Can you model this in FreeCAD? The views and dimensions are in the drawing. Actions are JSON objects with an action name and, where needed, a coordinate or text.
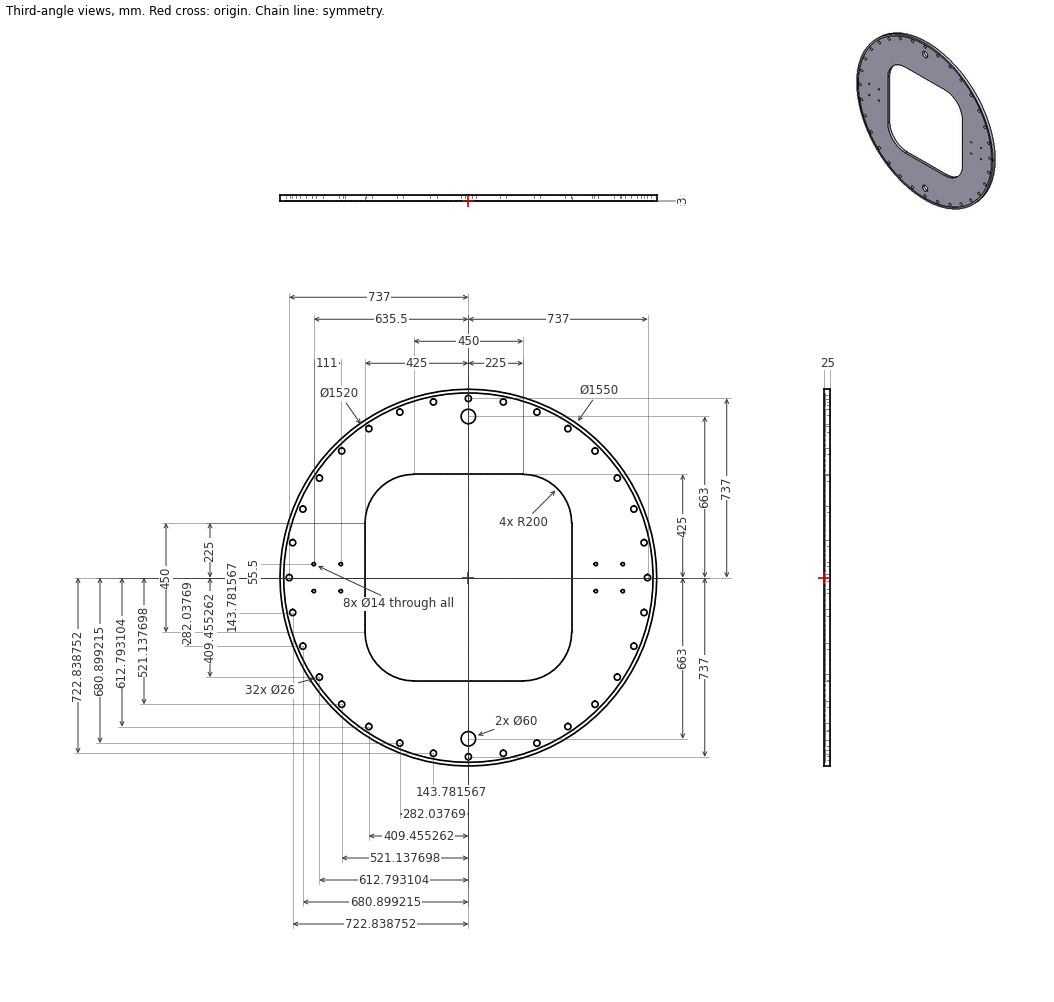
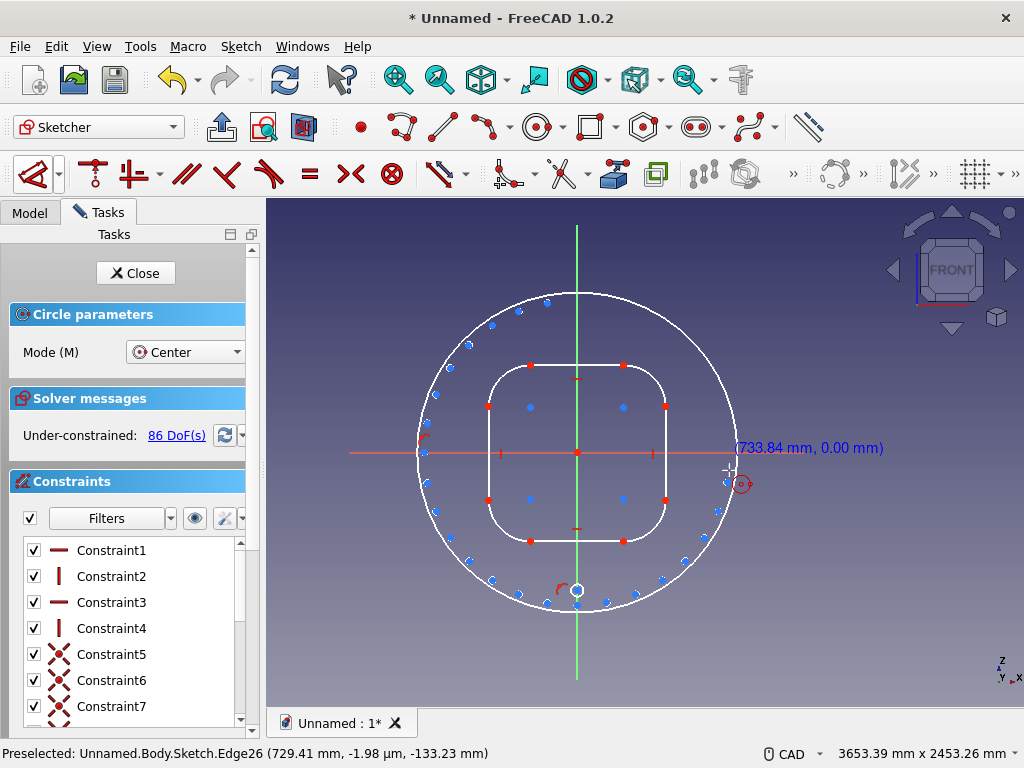
{"action": "scroll", "coordinate": [730, 453], "scroll_direction": "up", "scroll_amount": 4}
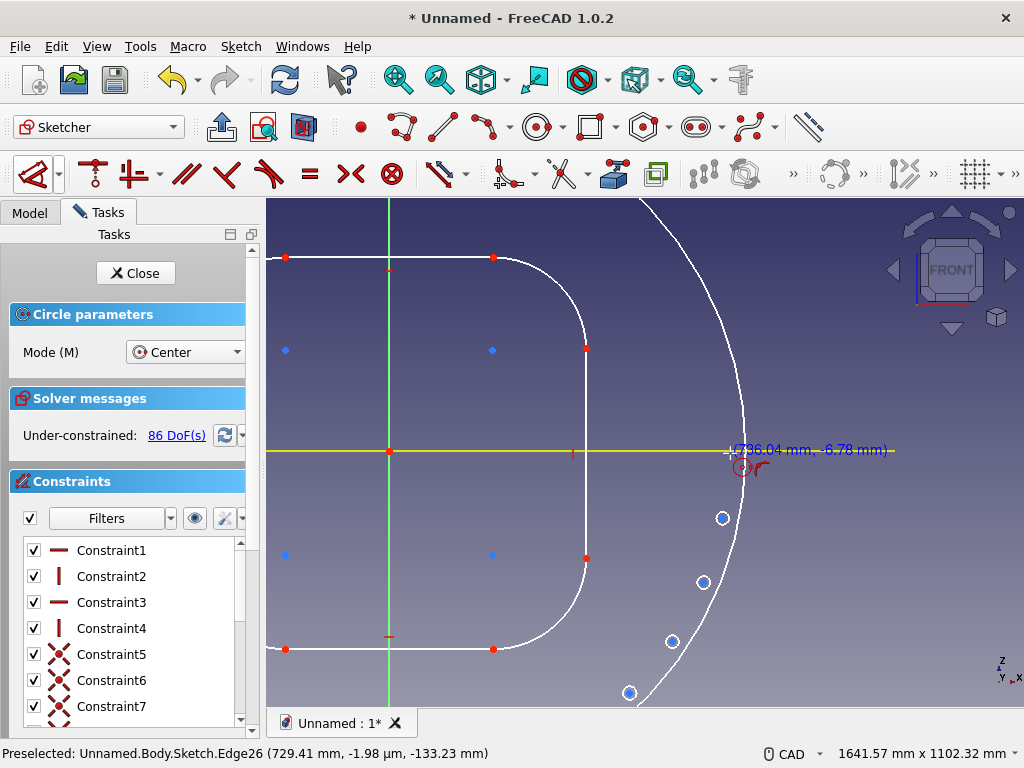
{"action": "left_click", "coordinate": [730, 451]}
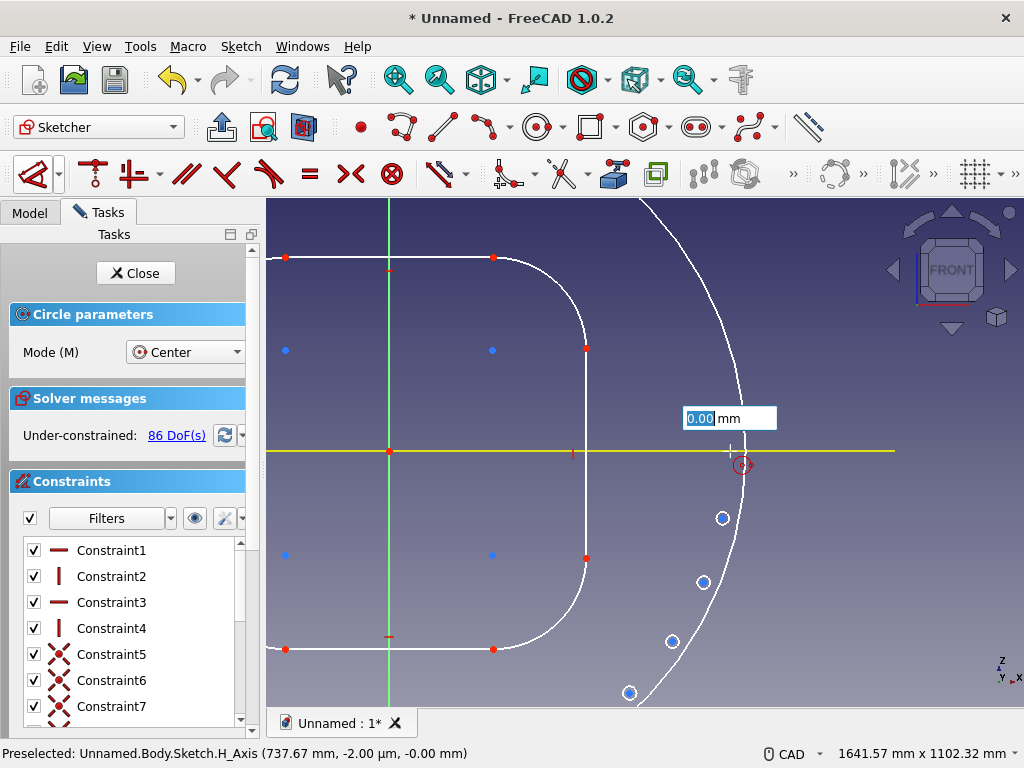
{"action": "scroll", "coordinate": [728, 457], "scroll_direction": "up", "scroll_amount": 6}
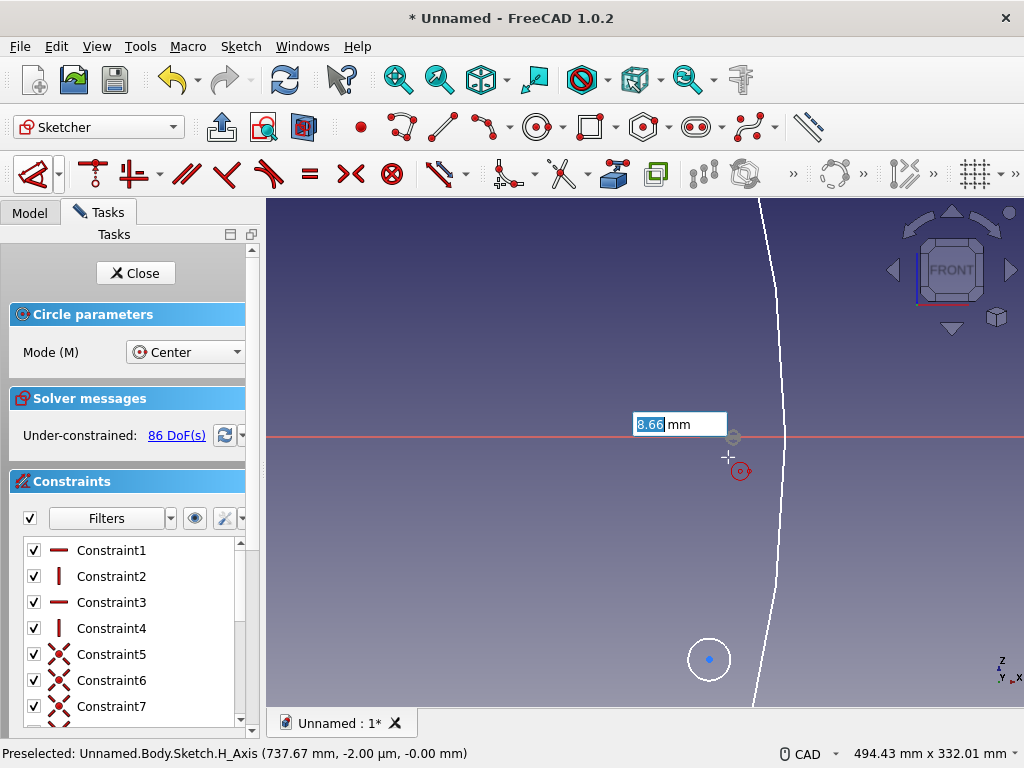
{"action": "left_click", "coordinate": [725, 456]}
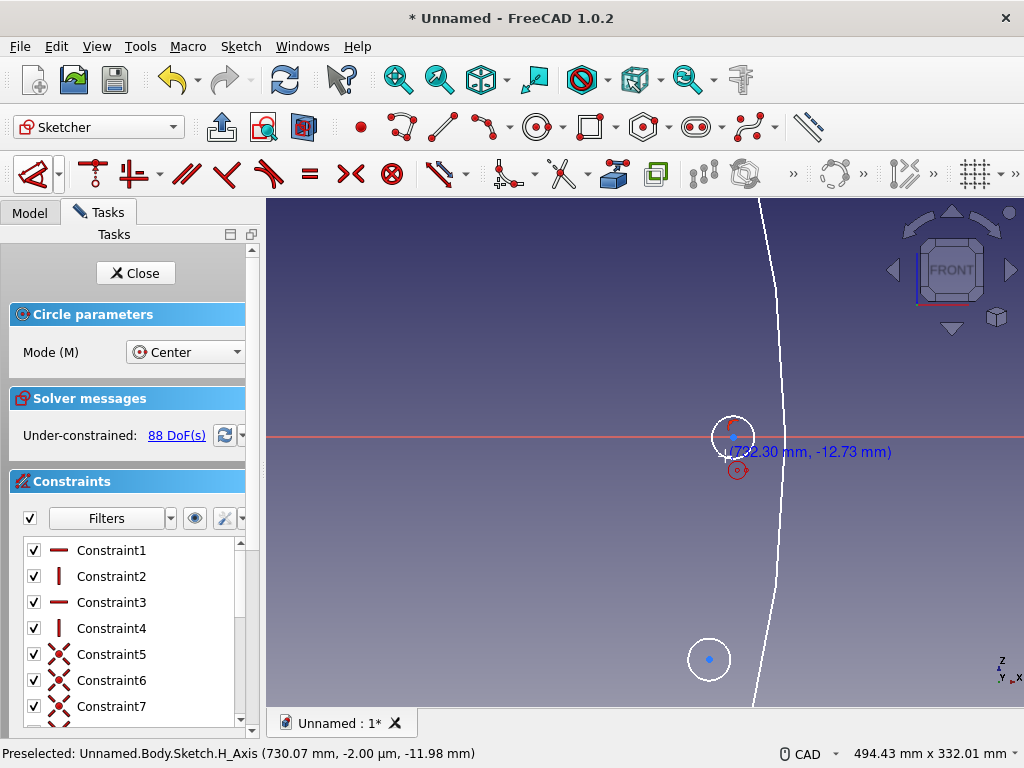
{"action": "scroll", "coordinate": [729, 455], "scroll_direction": "down", "scroll_amount": 10}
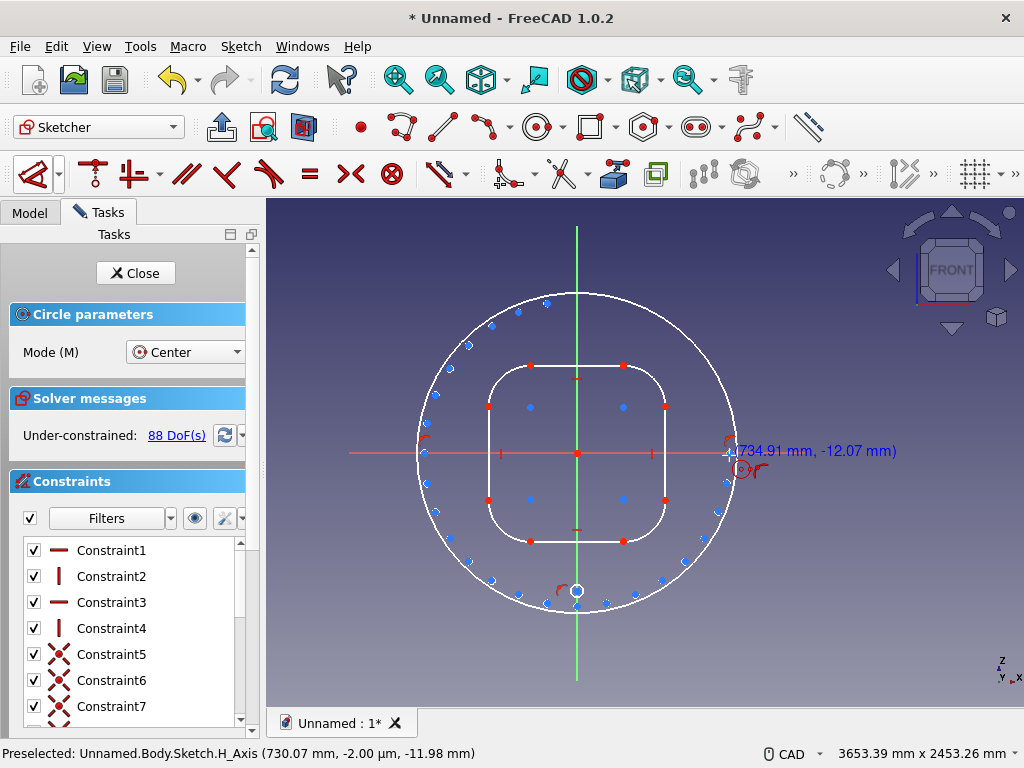
{"action": "scroll", "coordinate": [577, 316], "scroll_direction": "up", "scroll_amount": 7}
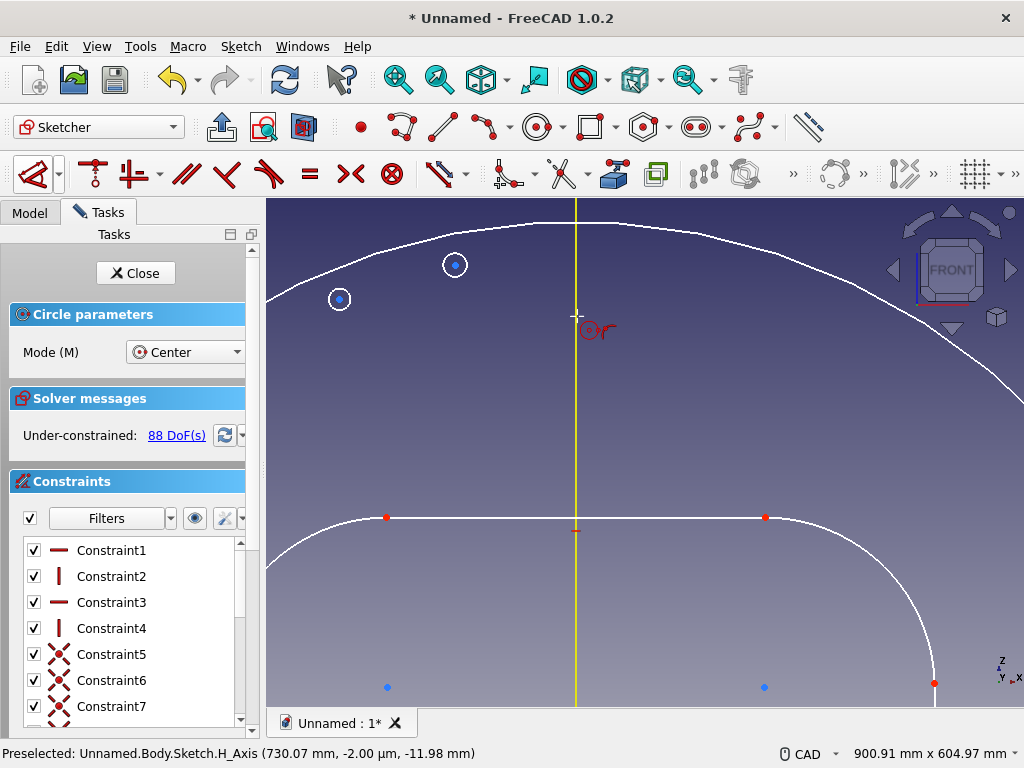
{"action": "left_click", "coordinate": [576, 313]}
{"action": "left_click", "coordinate": [594, 295]}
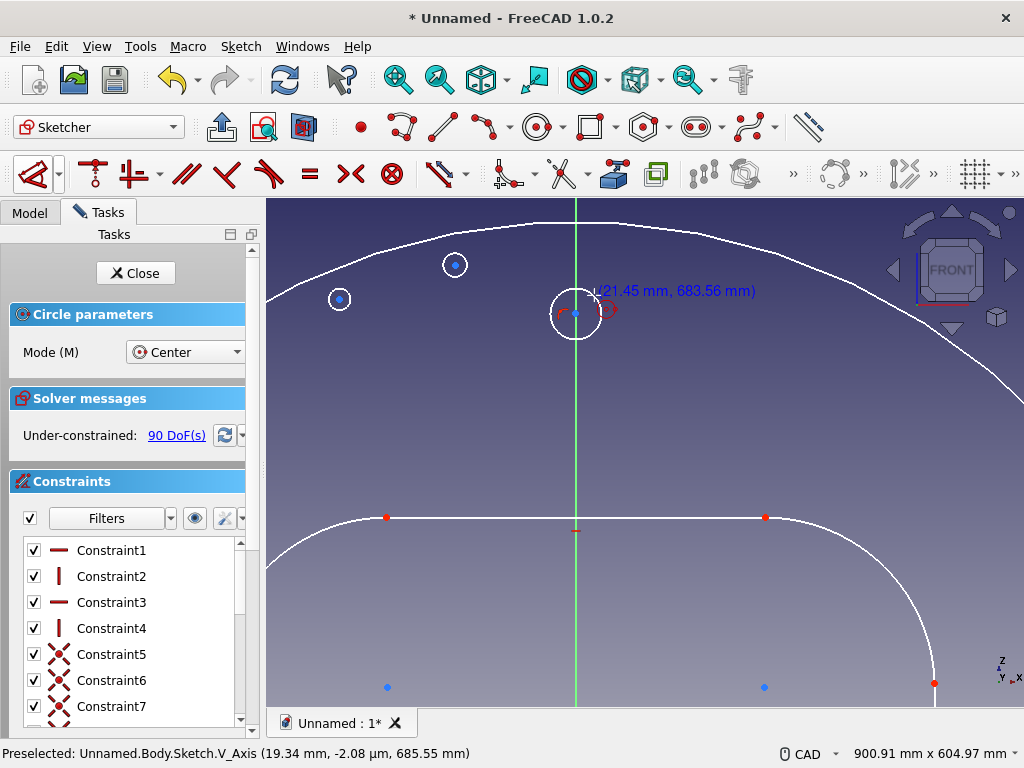
{"action": "scroll", "coordinate": [576, 251], "scroll_direction": "up", "scroll_amount": 4}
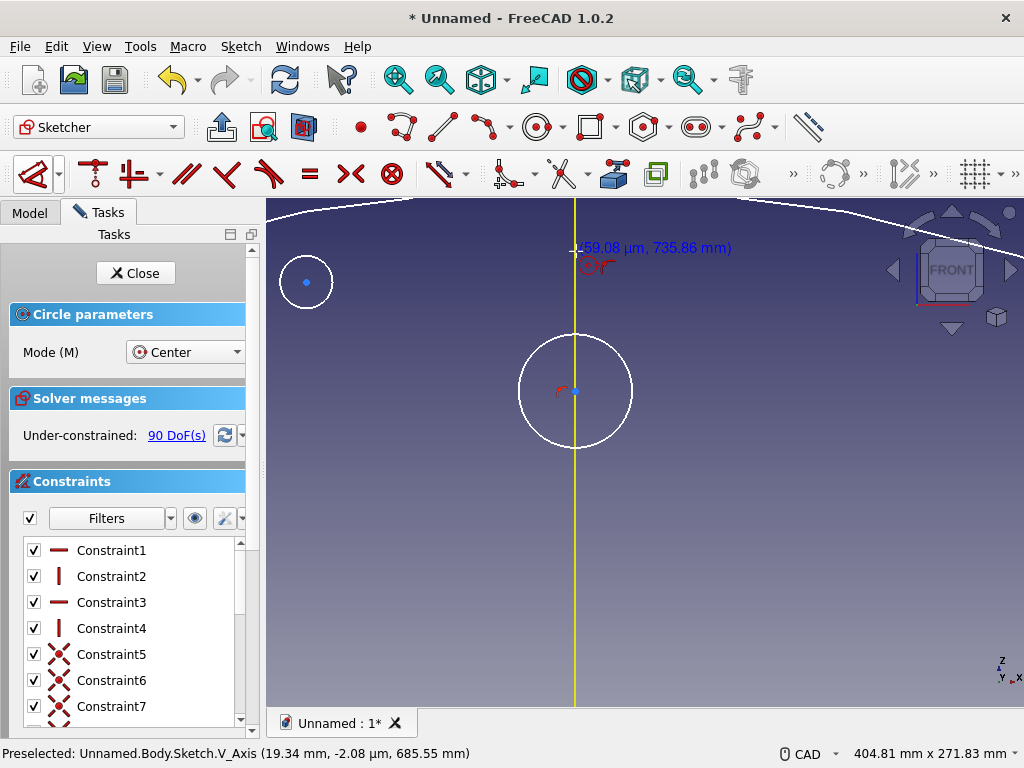
{"action": "scroll", "coordinate": [577, 306], "scroll_direction": "down", "scroll_amount": 11}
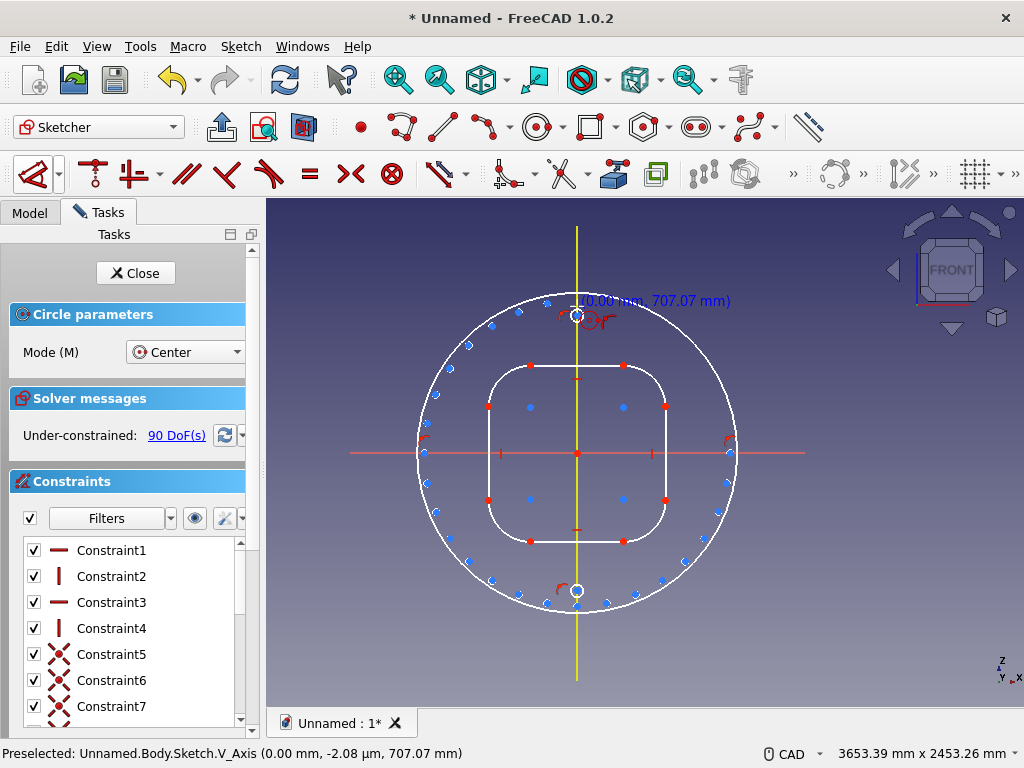
{"action": "scroll", "coordinate": [577, 300], "scroll_direction": "up", "scroll_amount": 4}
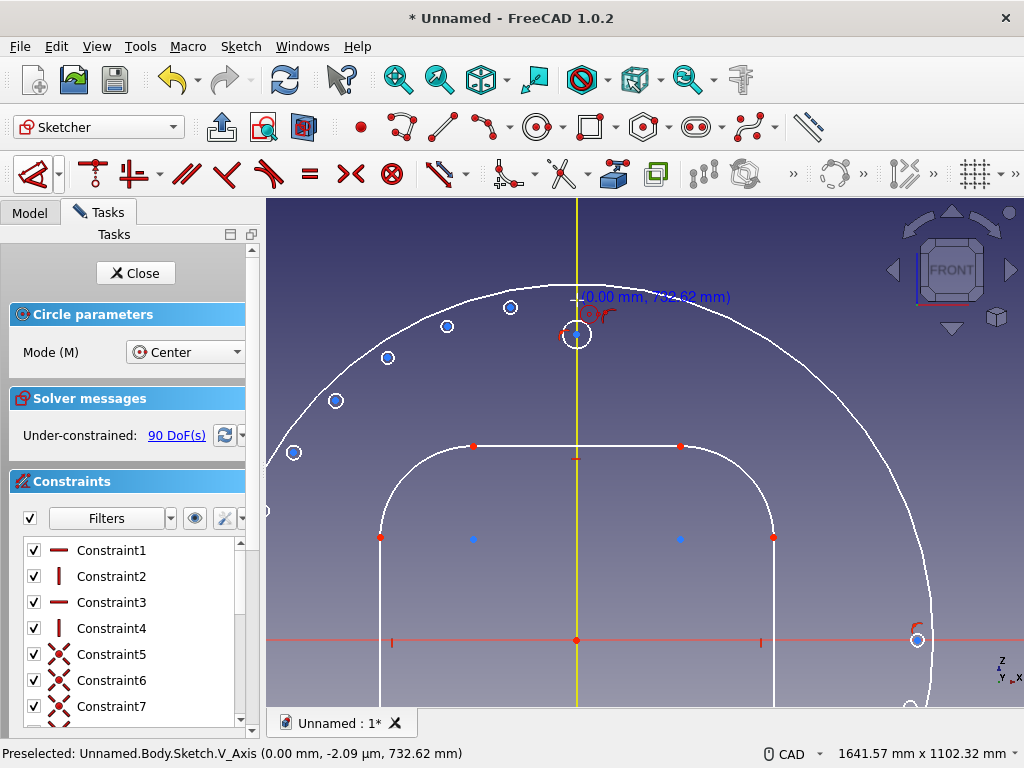
{"action": "left_click", "coordinate": [577, 300]}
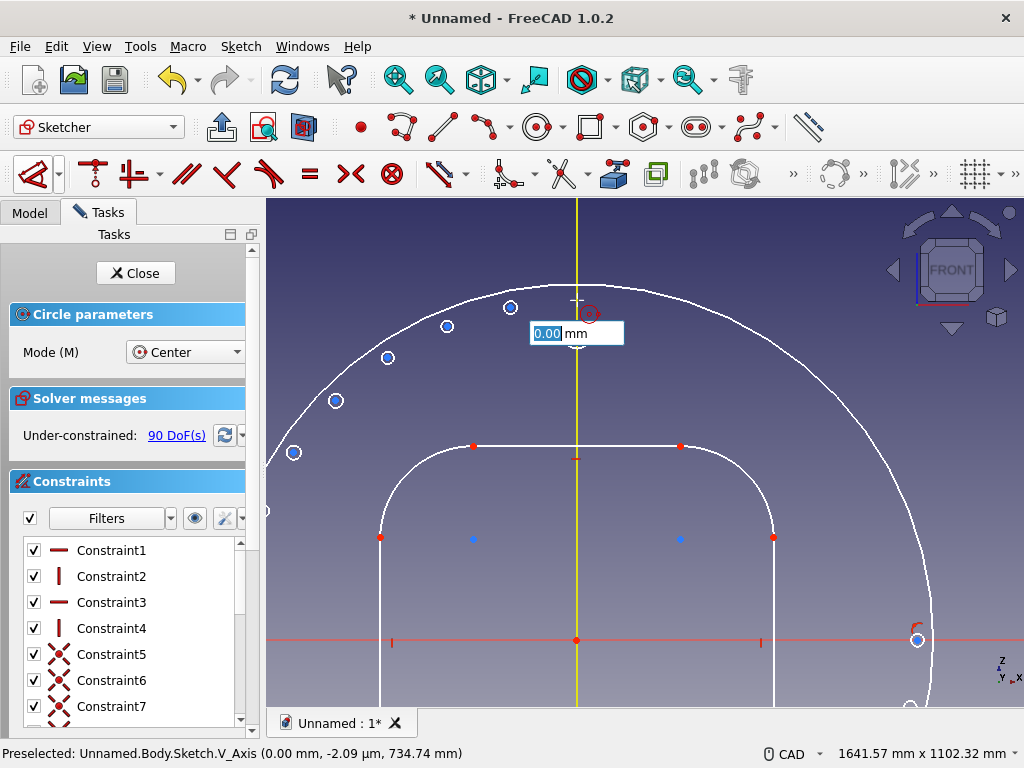
{"action": "scroll", "coordinate": [583, 298], "scroll_direction": "up", "scroll_amount": 6}